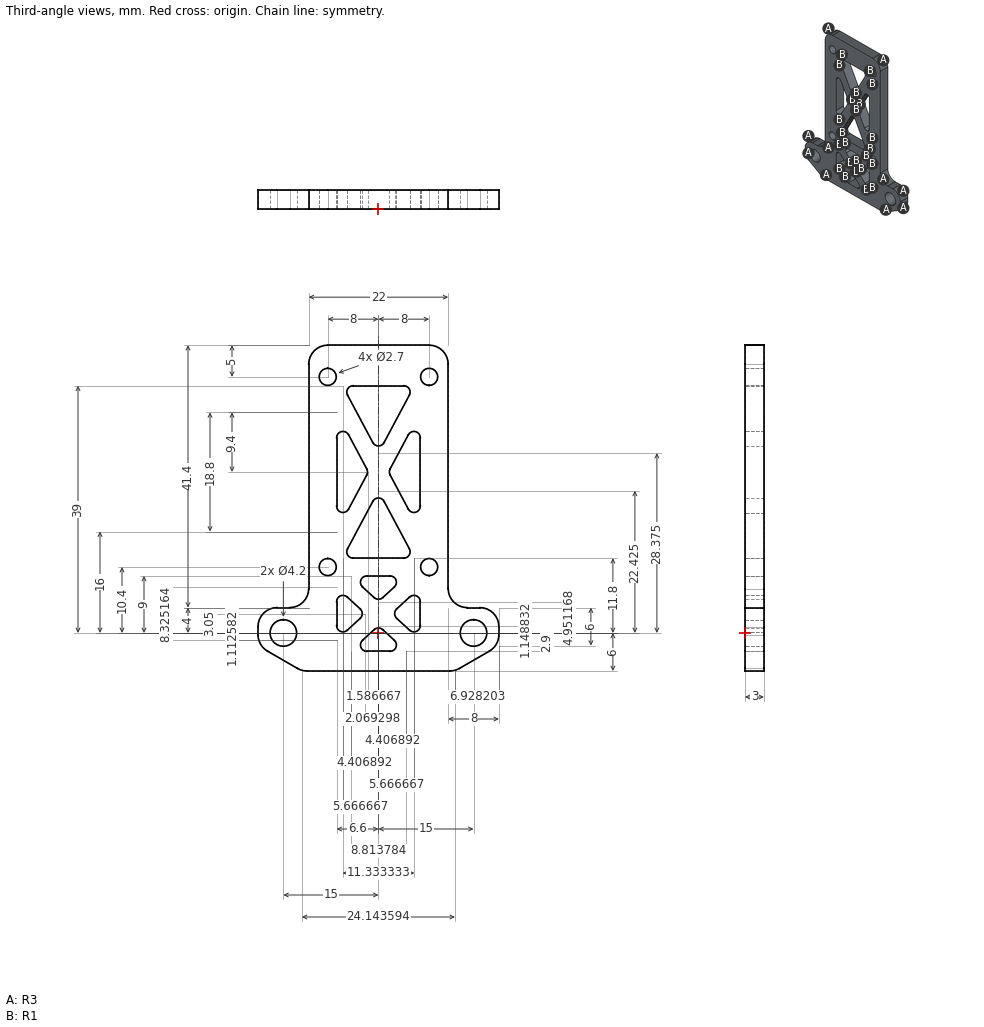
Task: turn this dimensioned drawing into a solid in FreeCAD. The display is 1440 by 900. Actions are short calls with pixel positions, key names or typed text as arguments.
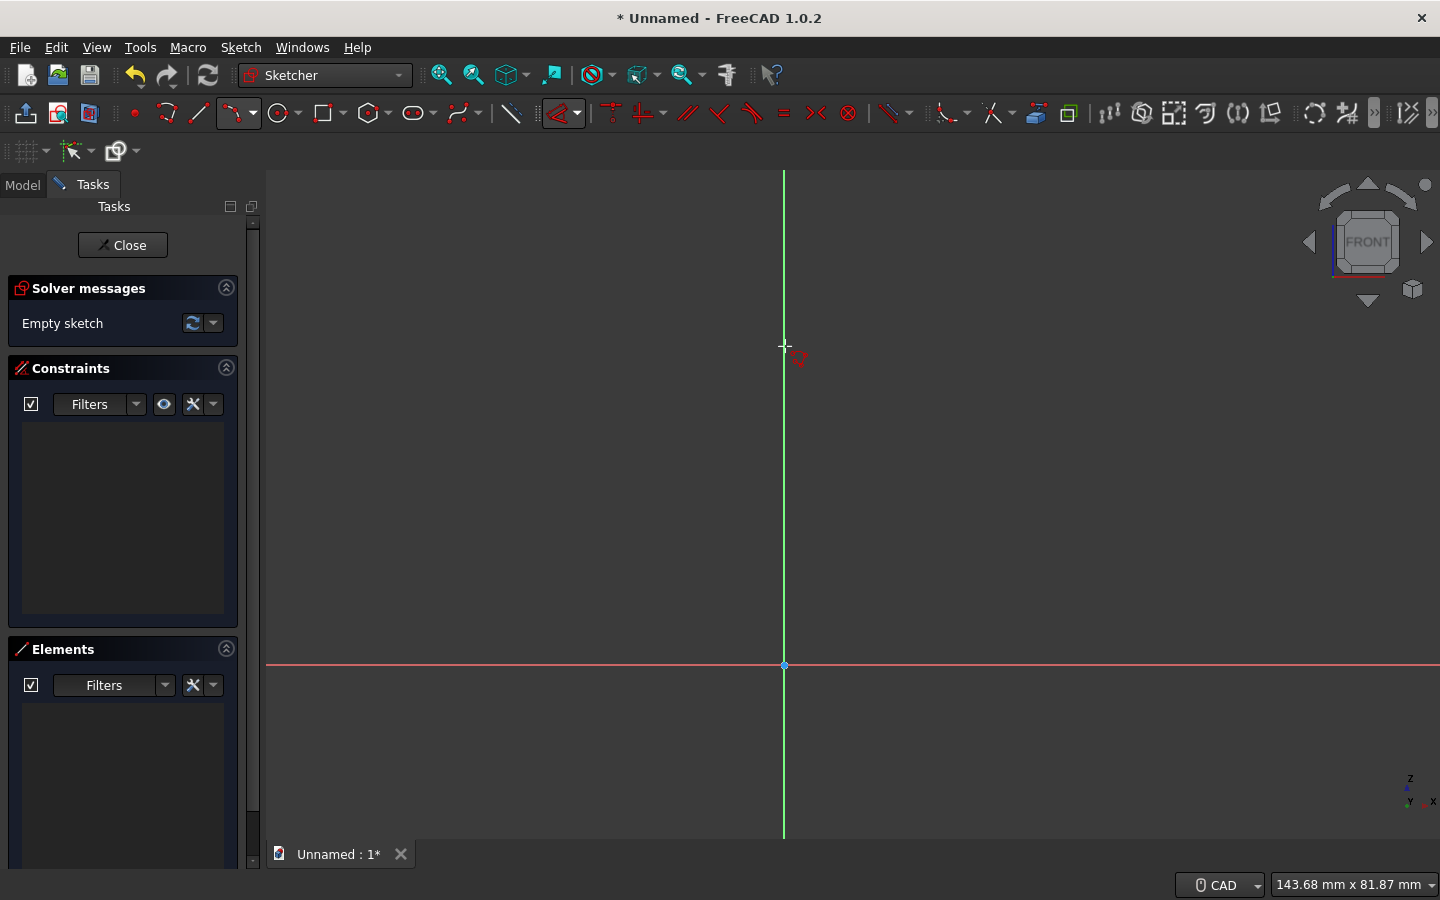
click(694, 633)
click(694, 294)
click(874, 294)
click(874, 633)
click(939, 633)
click(939, 682)
click(883, 714)
click(685, 714)
click(629, 682)
click(629, 633)
click(694, 634)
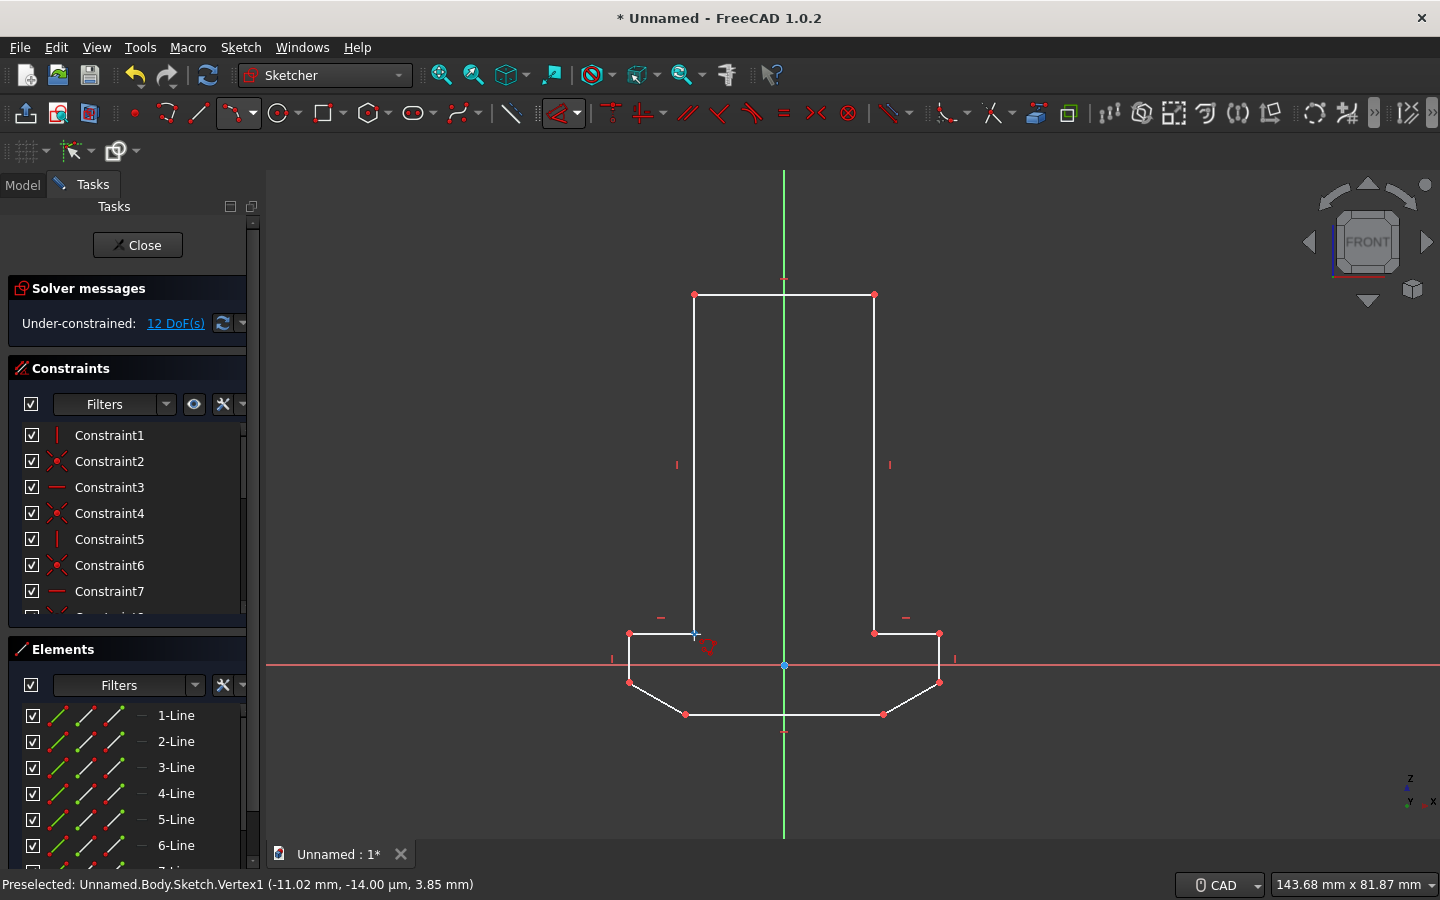
key(g)
key(c)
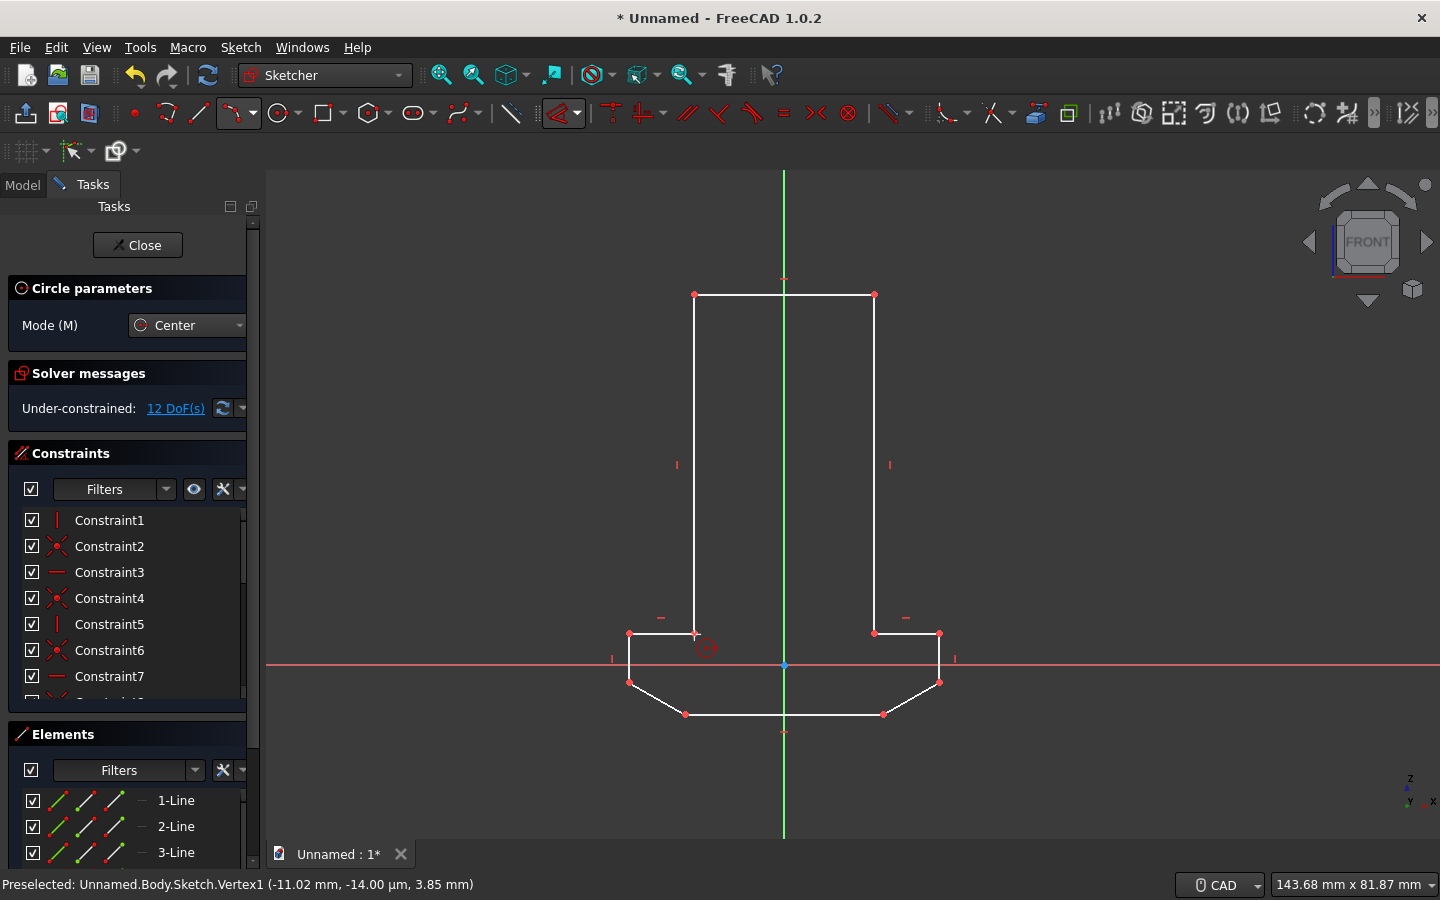
scroll(719, 335, up, 4)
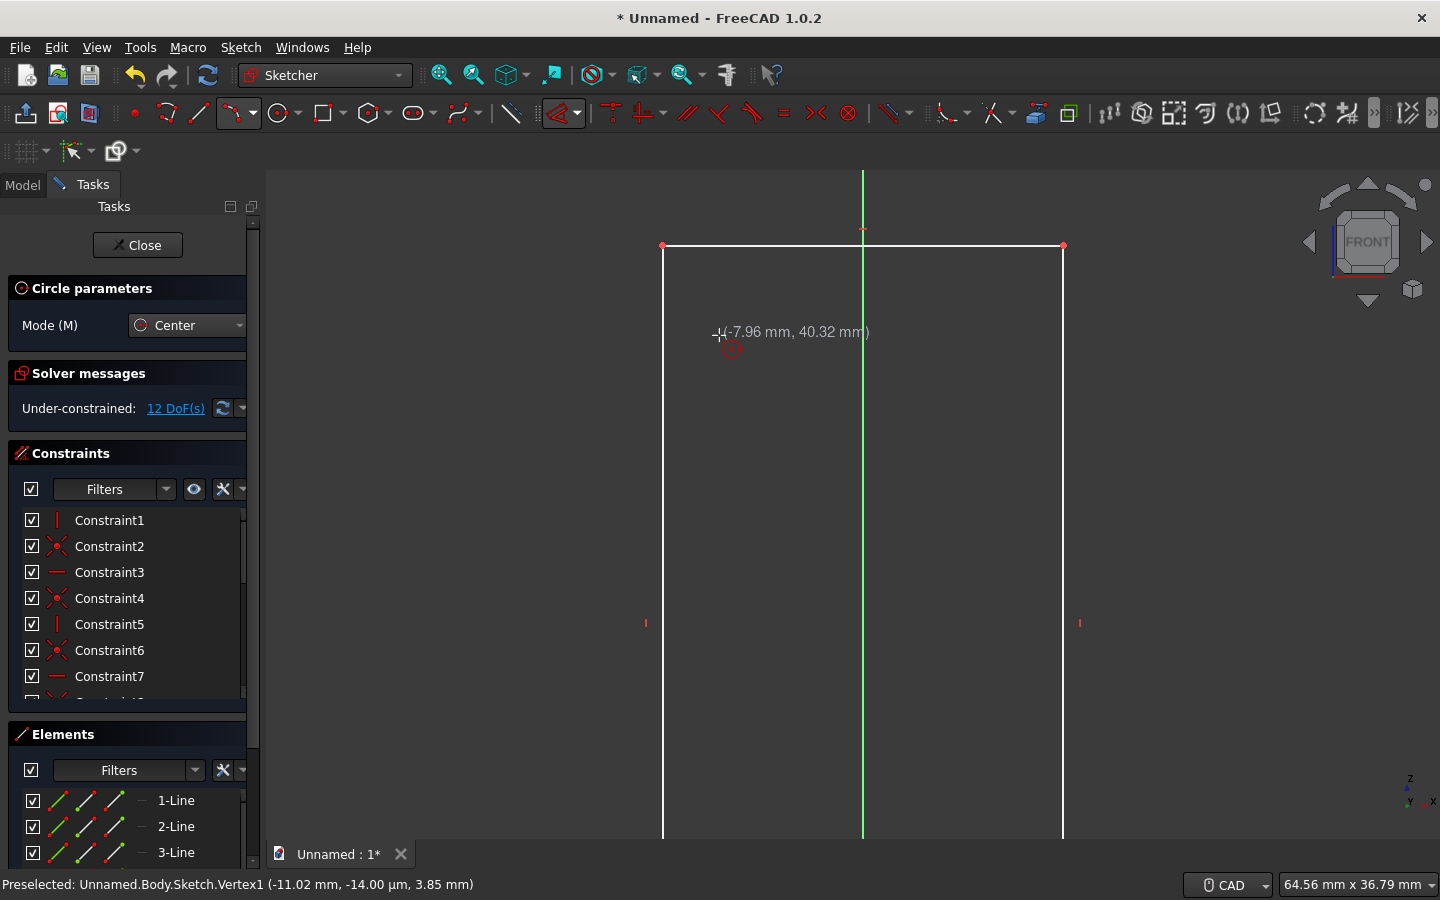
click(718, 335)
click(735, 318)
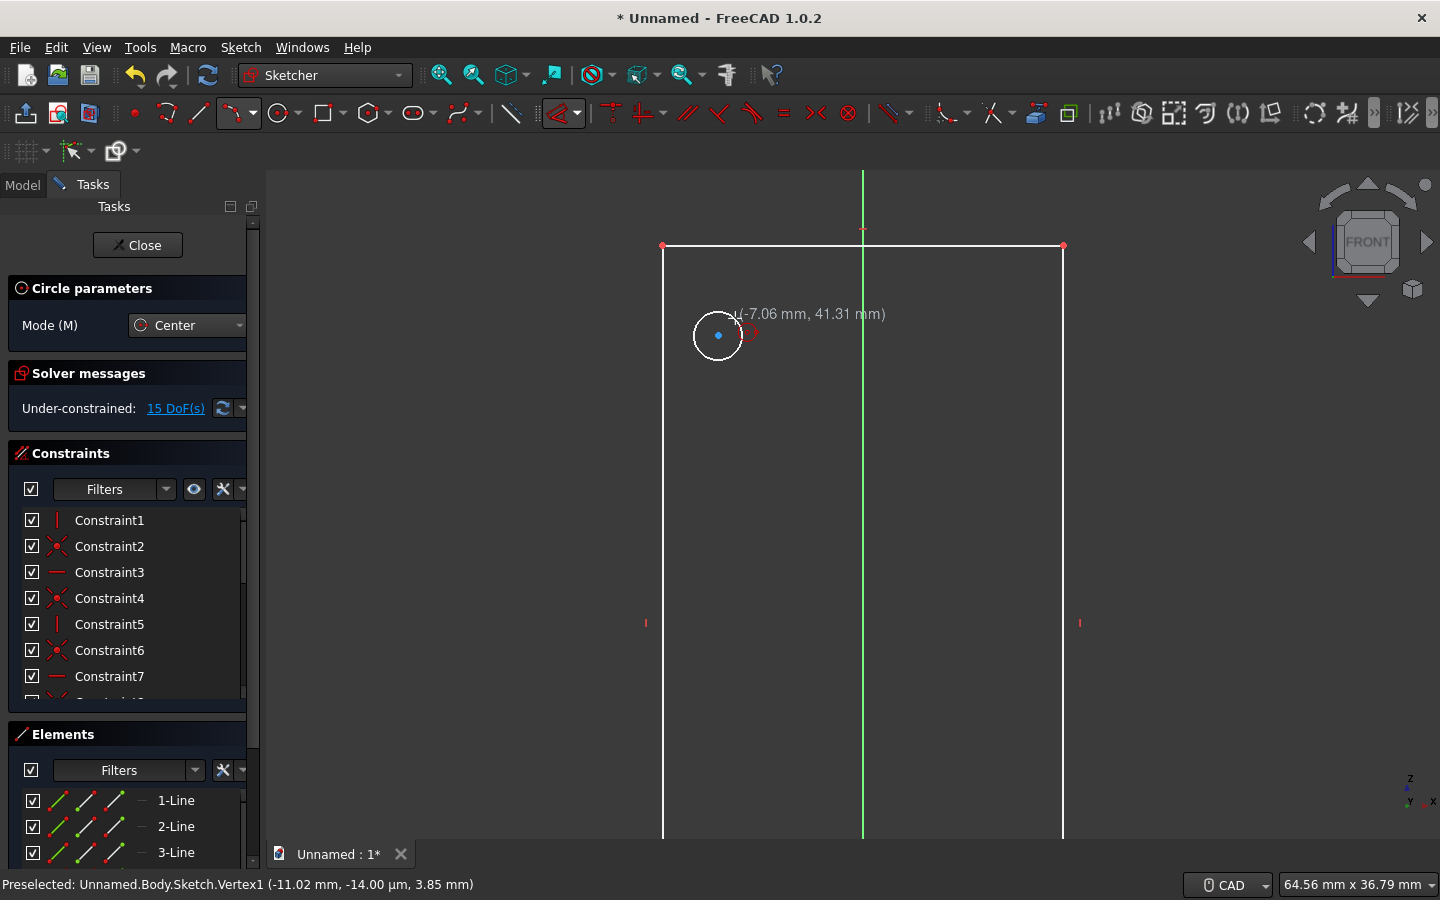
click(1009, 335)
click(1026, 318)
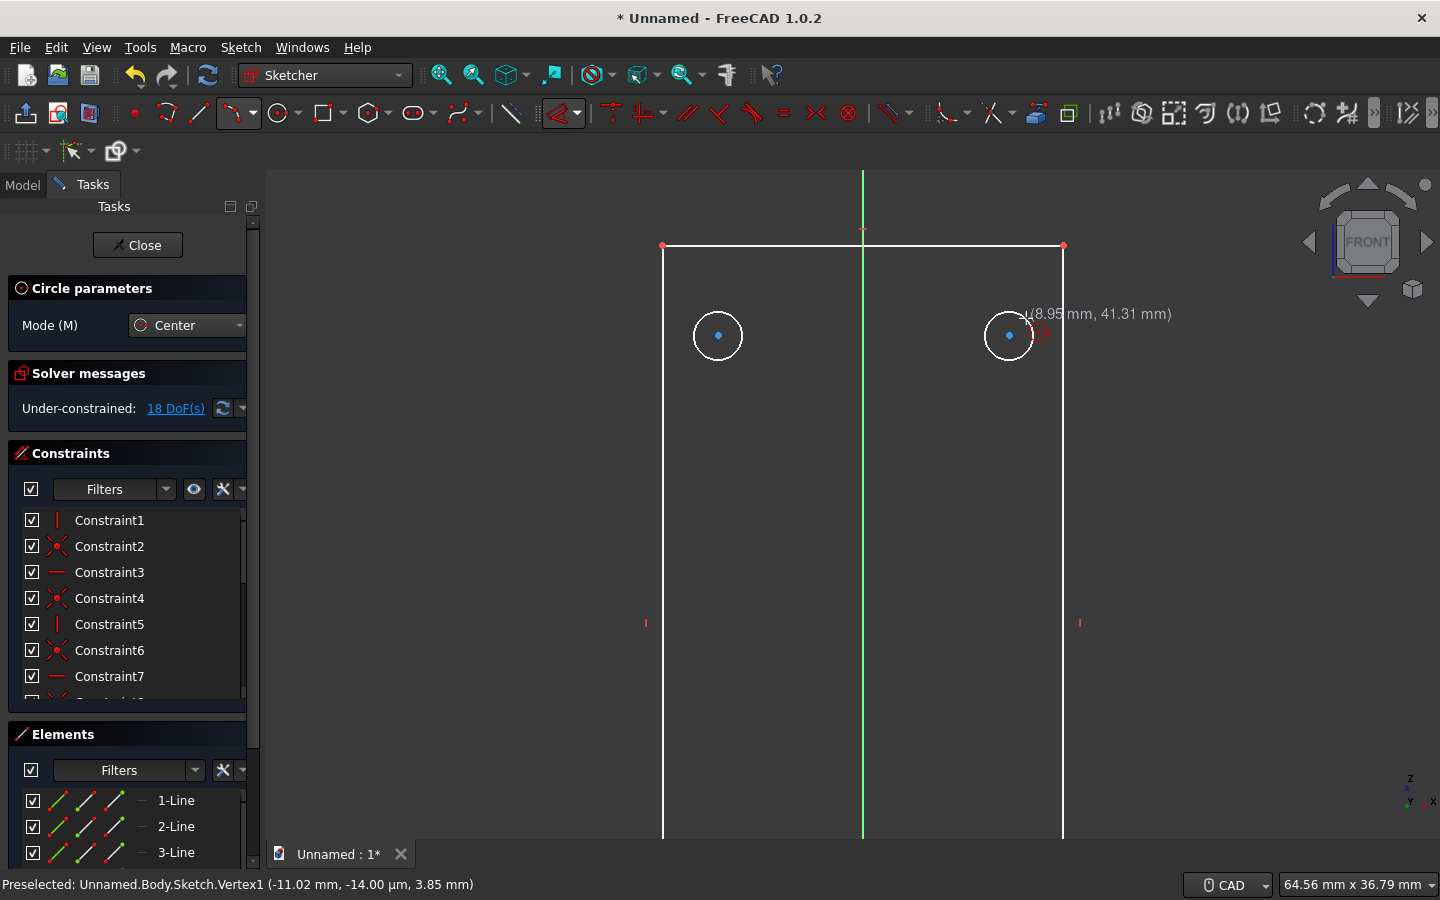
scroll(720, 335, down, 4)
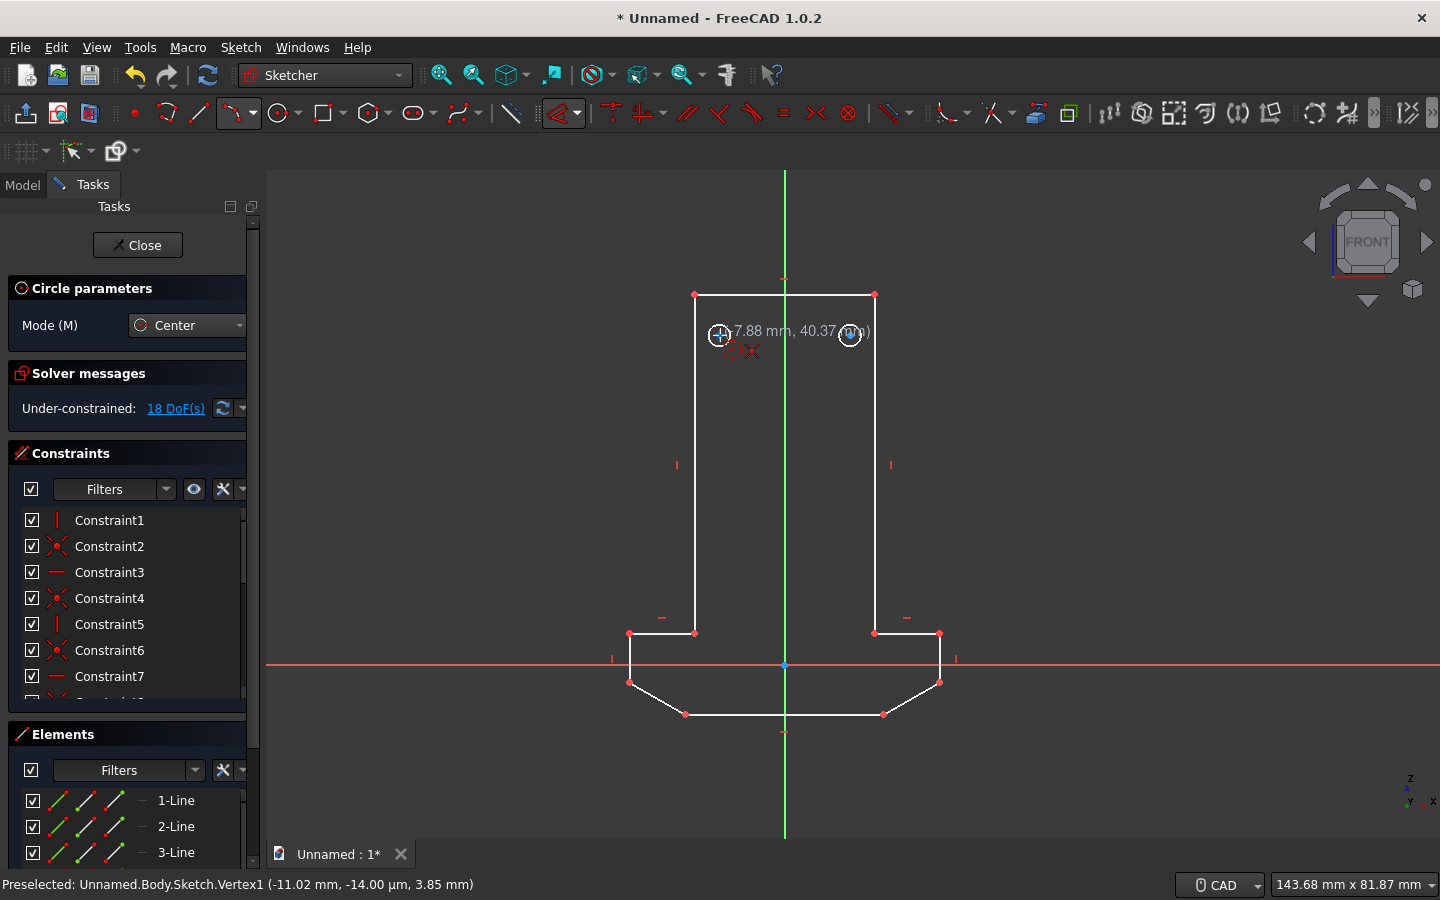
scroll(719, 580, up, 4)